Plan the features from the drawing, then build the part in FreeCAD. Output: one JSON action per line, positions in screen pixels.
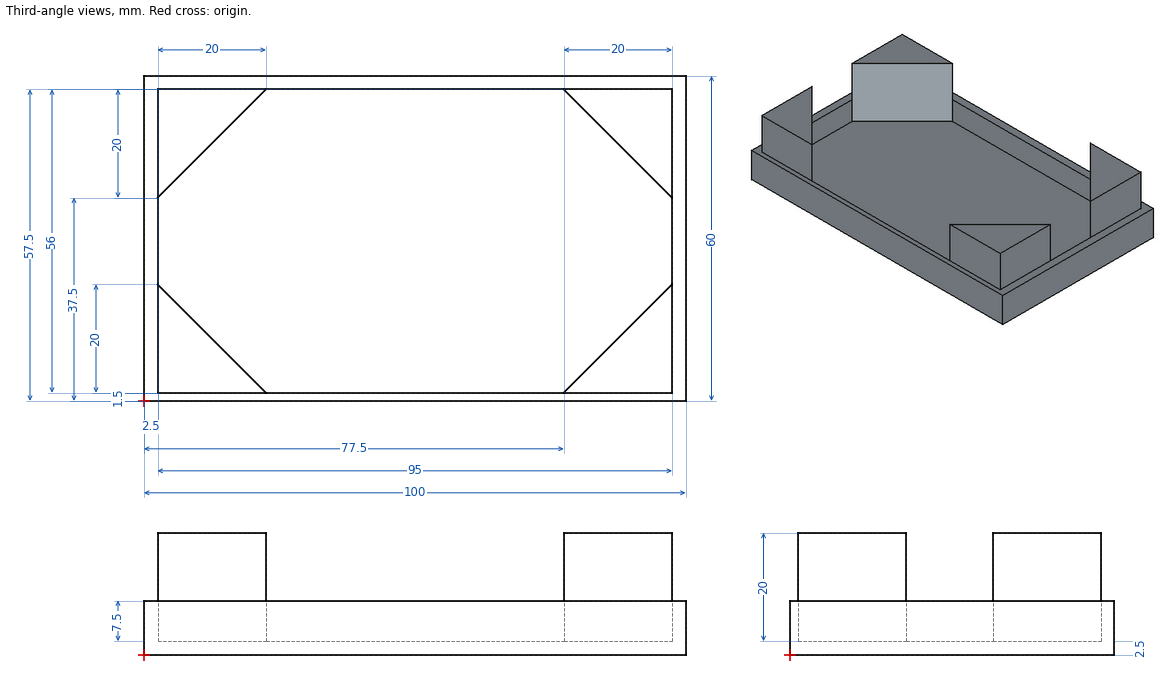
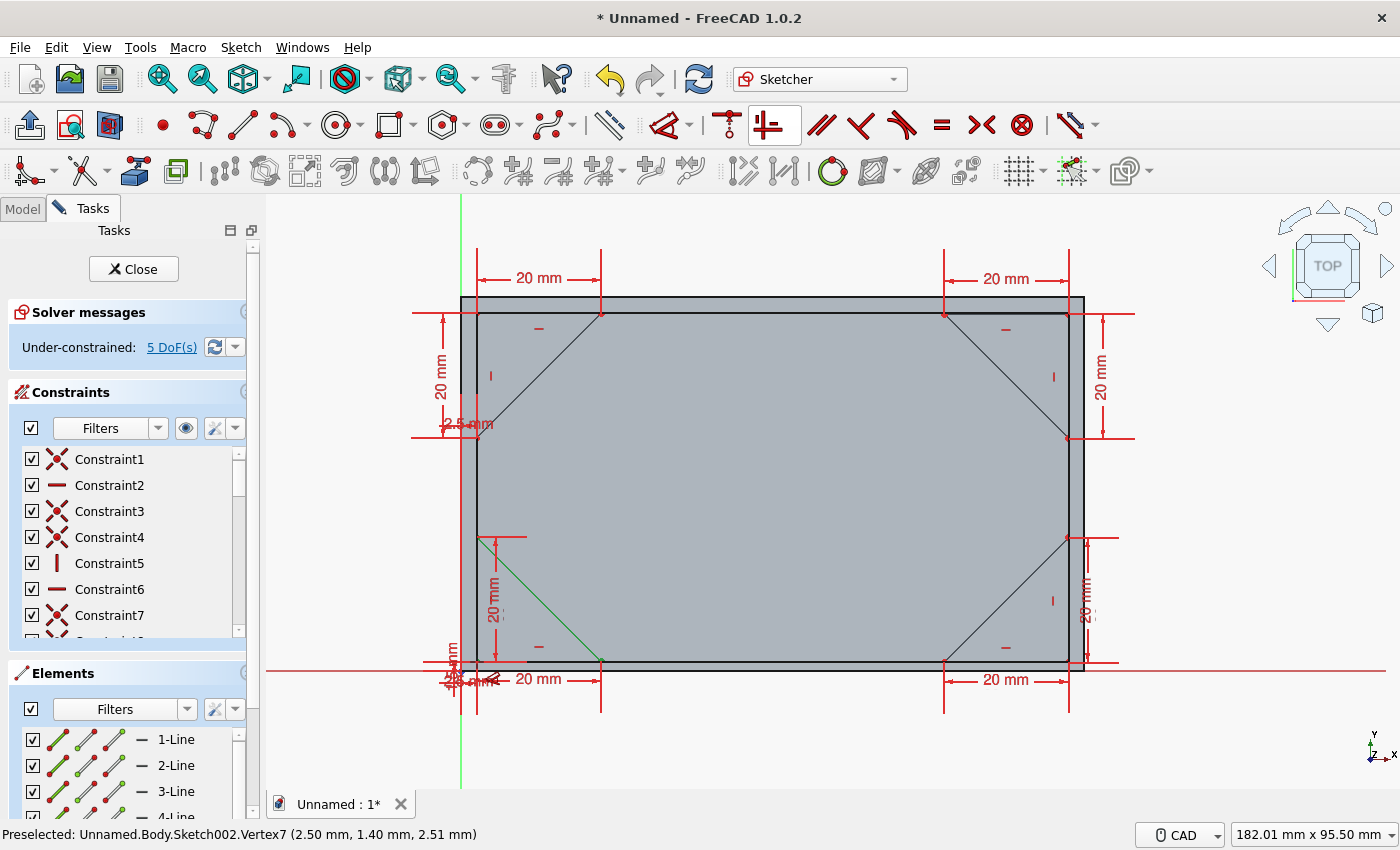
{"action": "scroll", "coordinate": [944, 663], "scroll_direction": "up", "scroll_amount": 8}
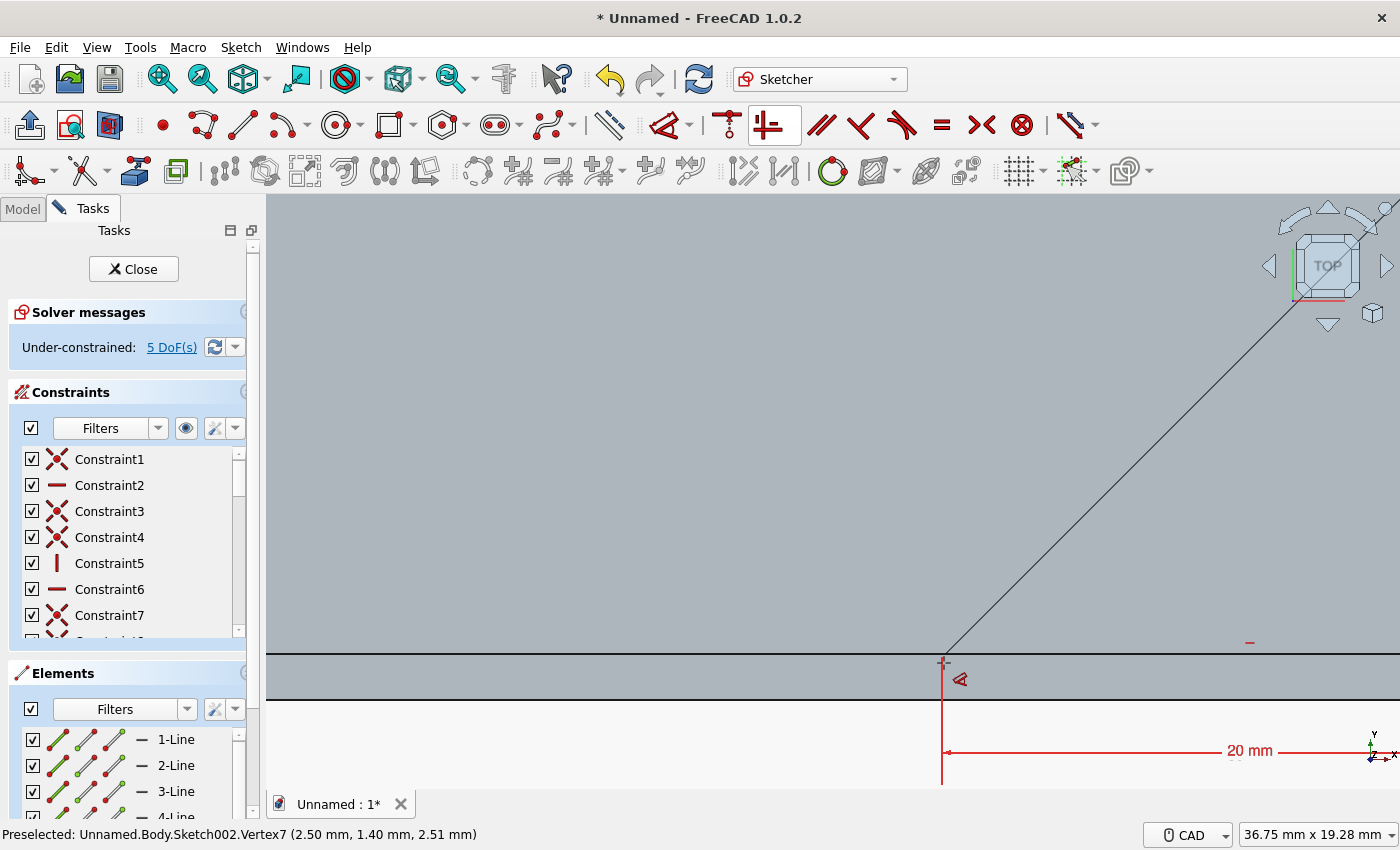
{"action": "left_click", "coordinate": [942, 658]}
{"action": "left_click", "coordinate": [976, 679]}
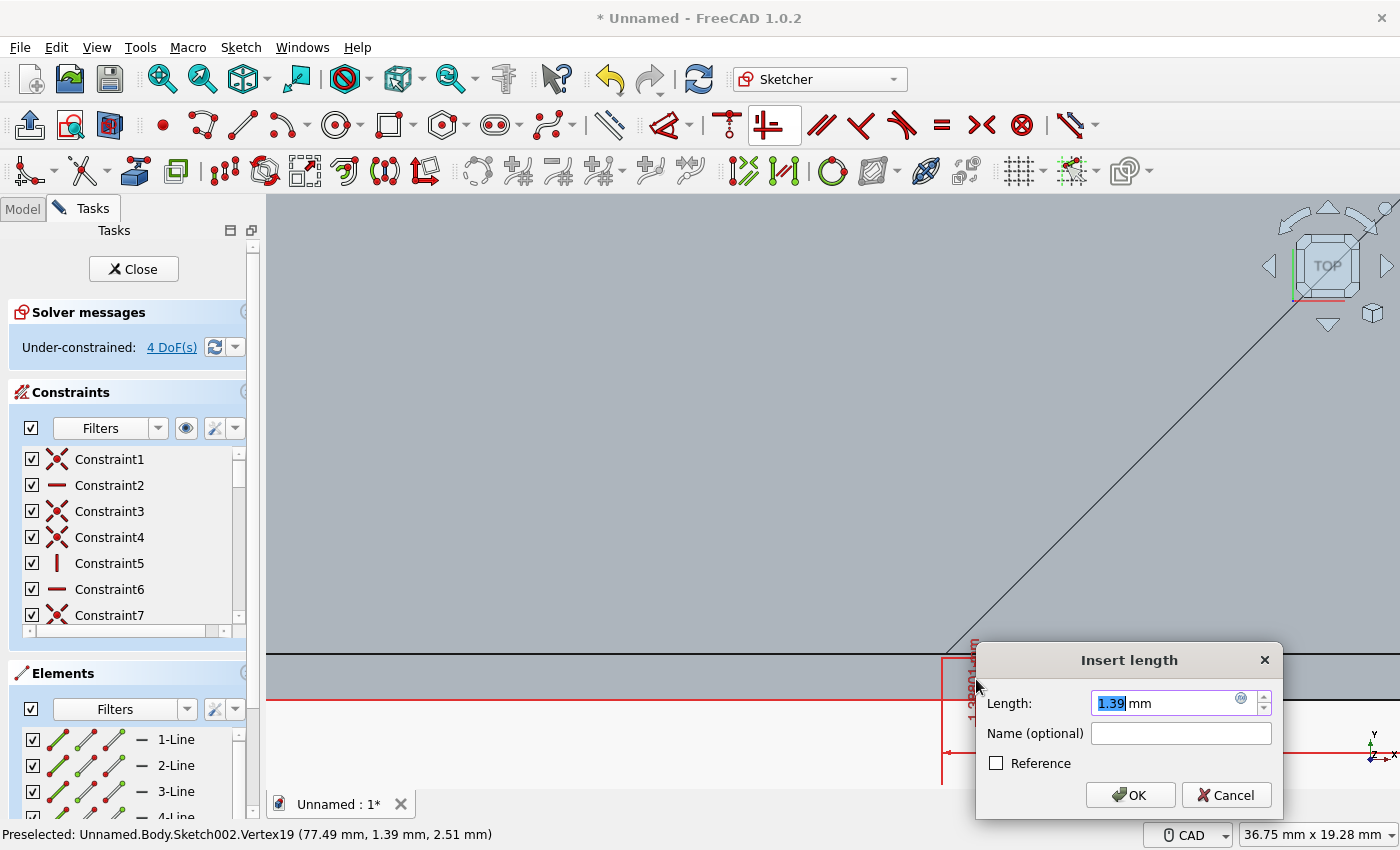
{"action": "type", "text": "1.5"}
{"action": "key", "text": "Return"}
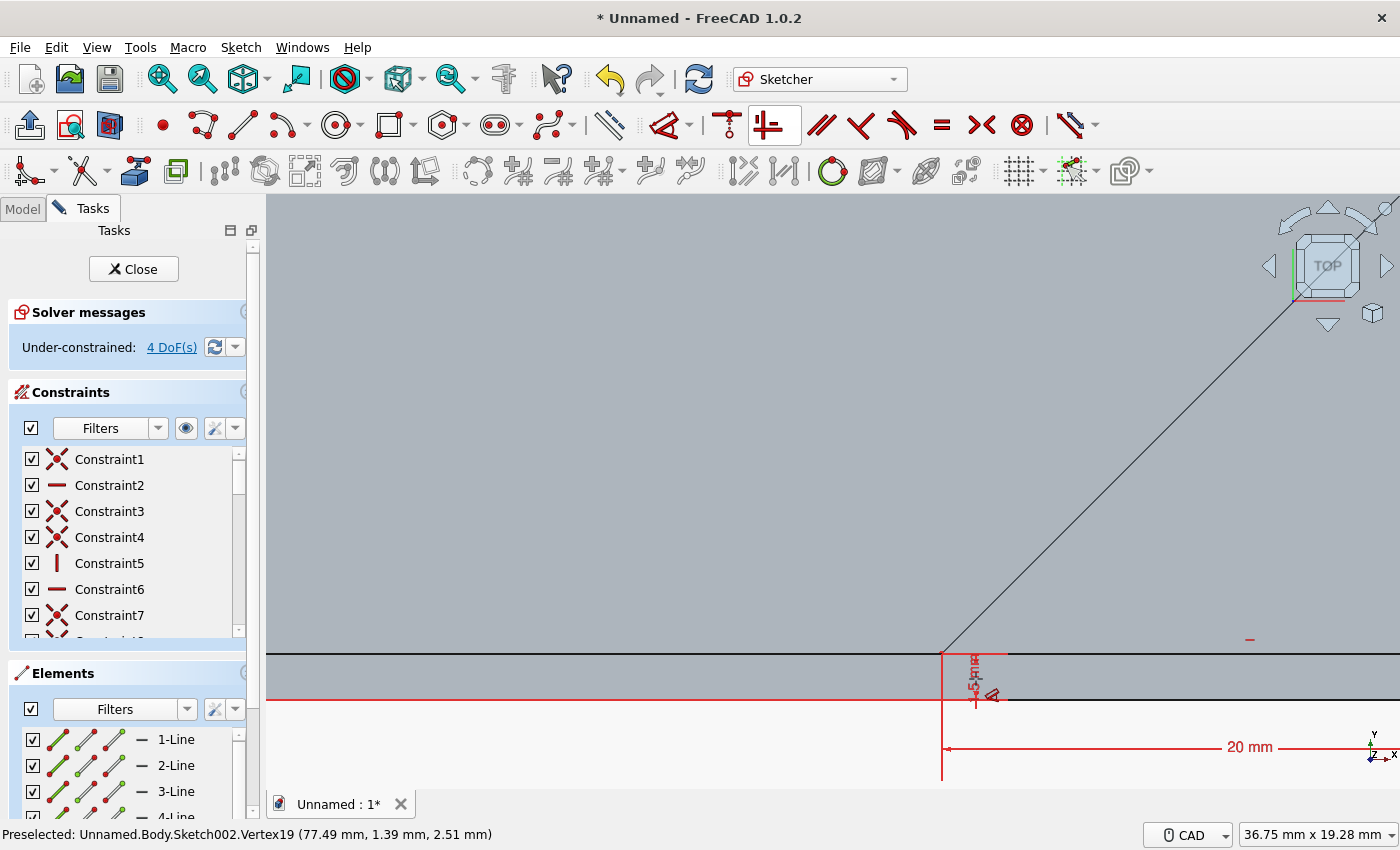
{"action": "scroll", "coordinate": [944, 663], "scroll_direction": "down", "scroll_amount": 8}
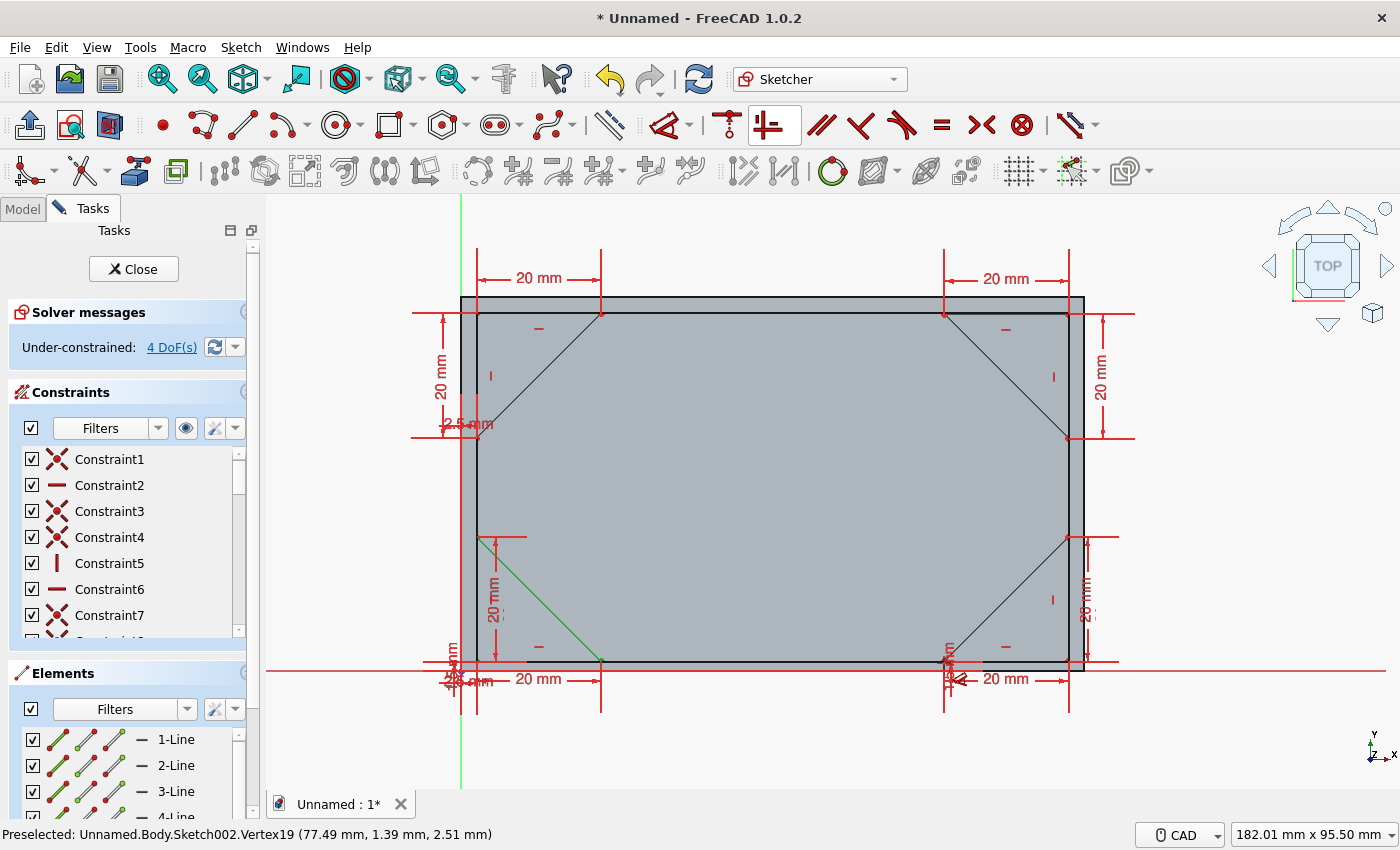
{"action": "left_click", "coordinate": [477, 438]}
{"action": "left_click", "coordinate": [427, 555]}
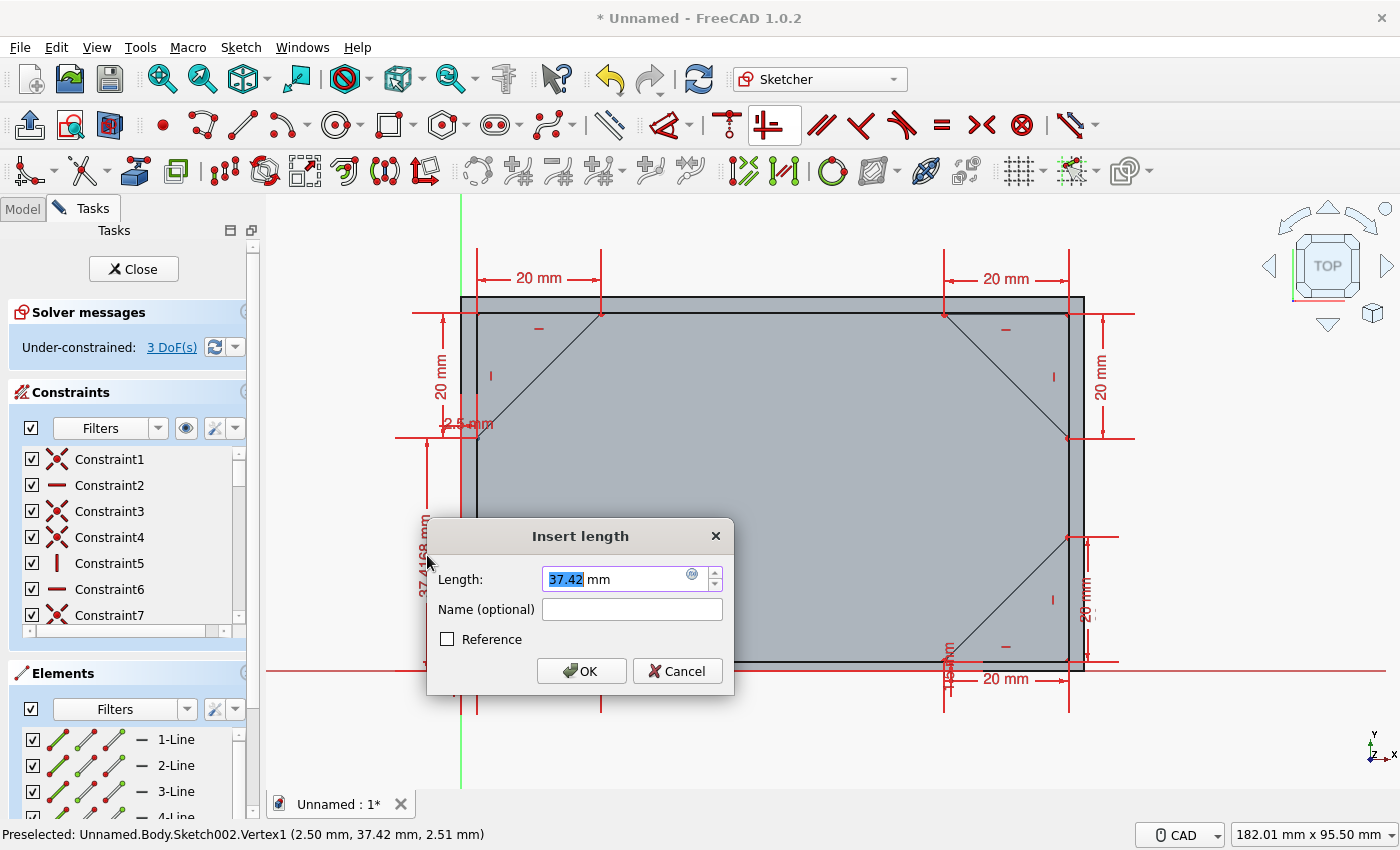
{"action": "type", "text": "37.5"}
{"action": "key", "text": "Return"}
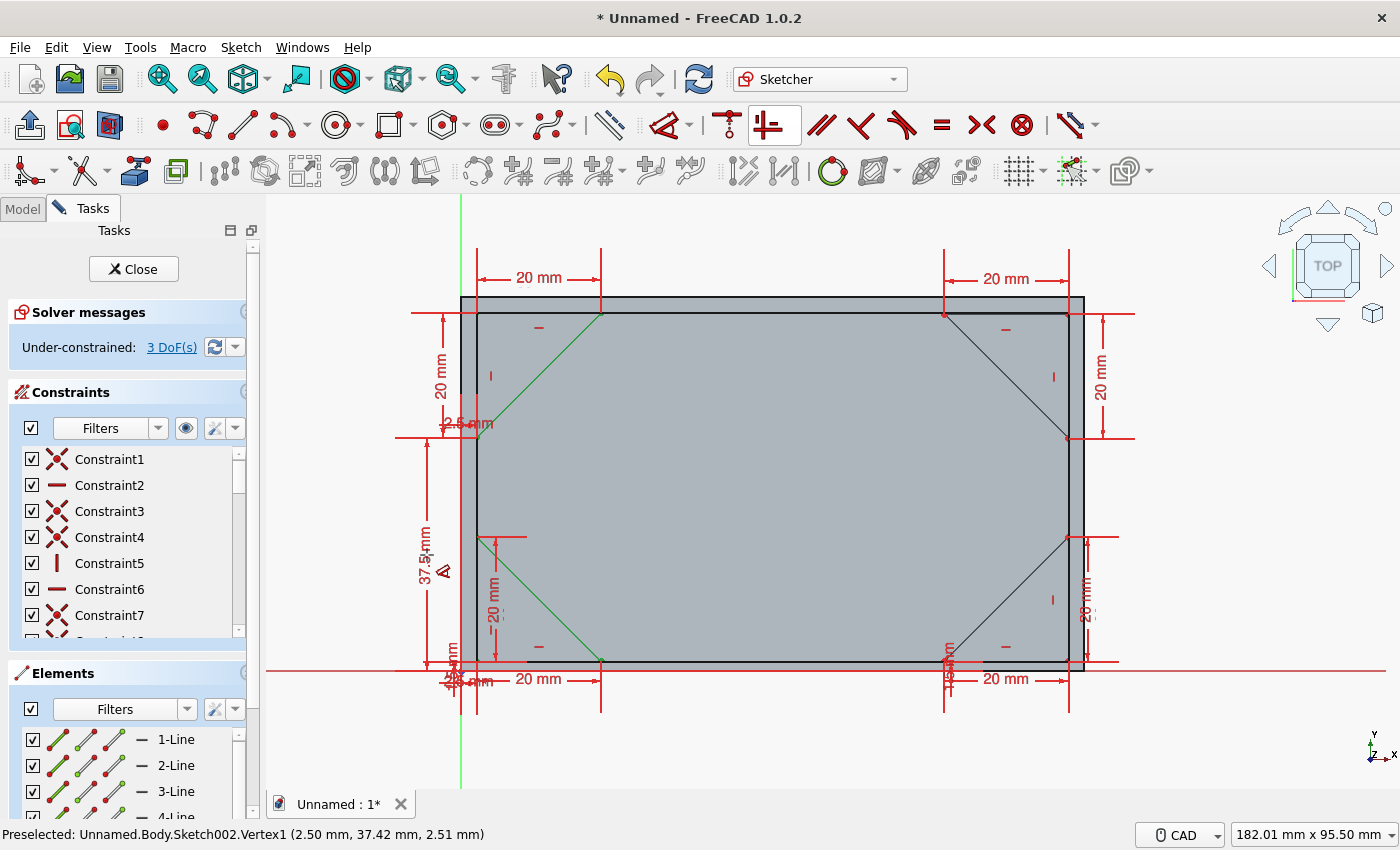
{"action": "left_click", "coordinate": [944, 314]}
{"action": "left_click", "coordinate": [703, 705]}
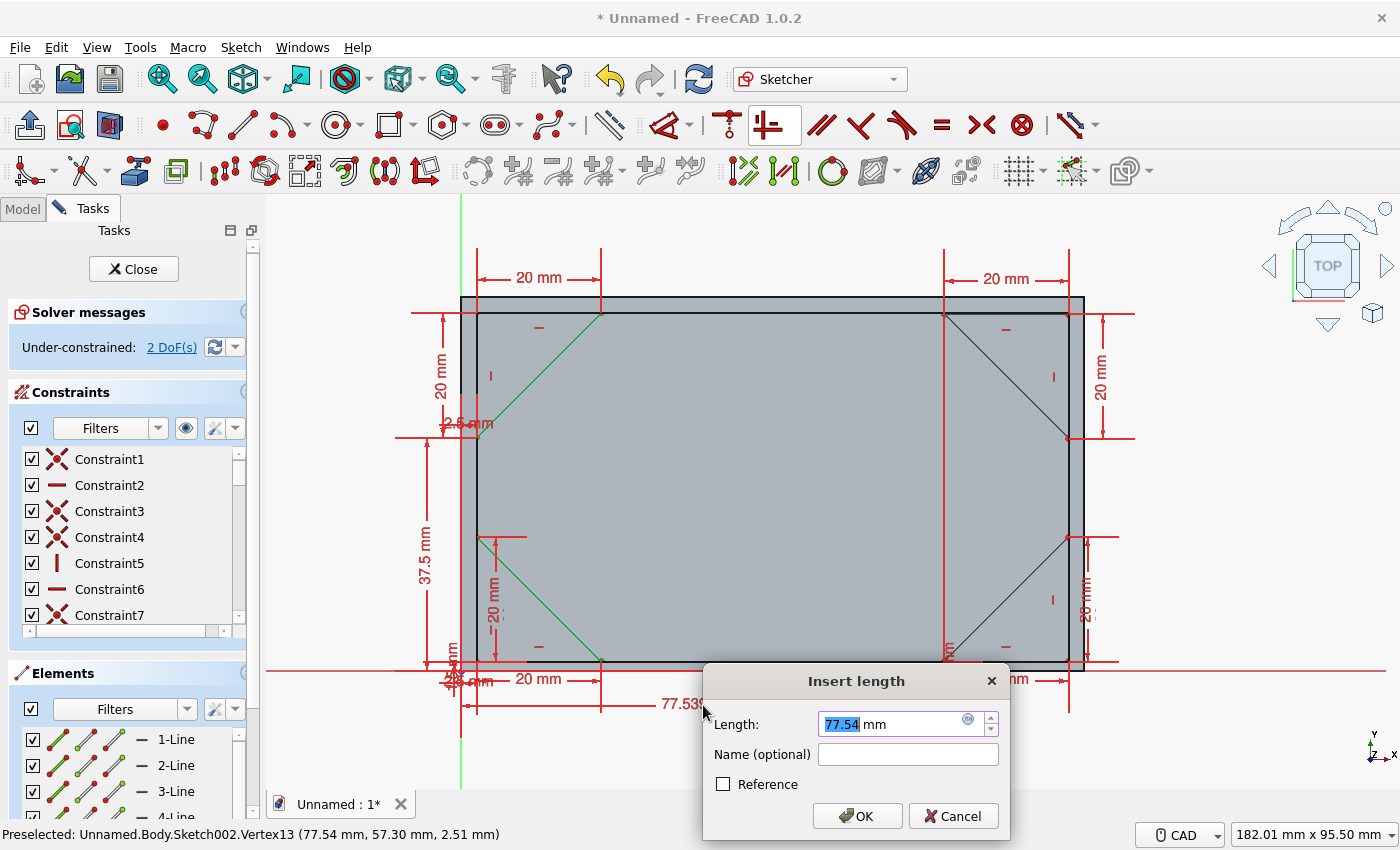
{"action": "type", "text": "77.5"}
{"action": "key", "text": "Return"}